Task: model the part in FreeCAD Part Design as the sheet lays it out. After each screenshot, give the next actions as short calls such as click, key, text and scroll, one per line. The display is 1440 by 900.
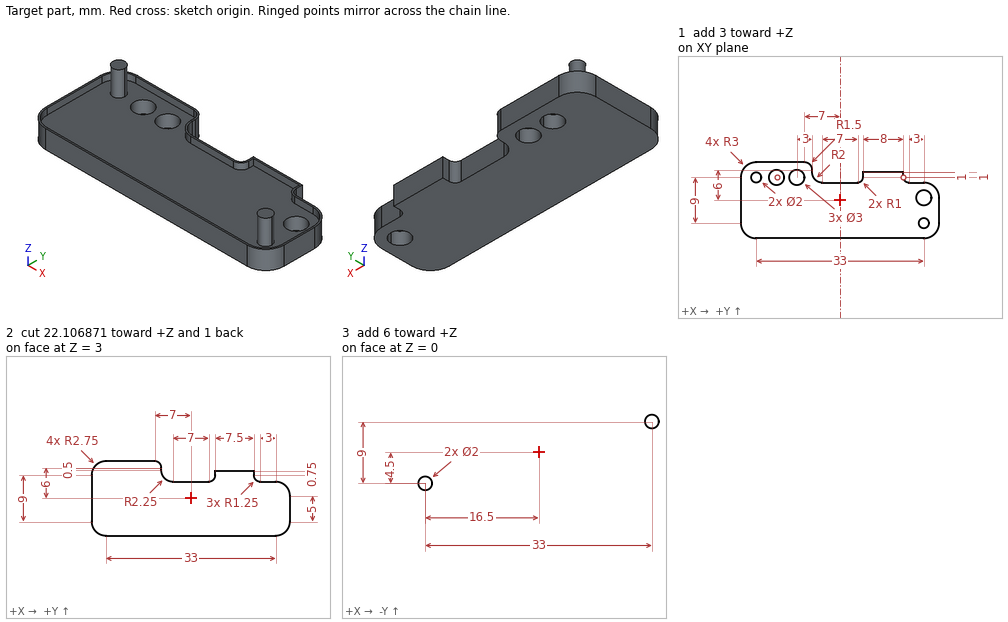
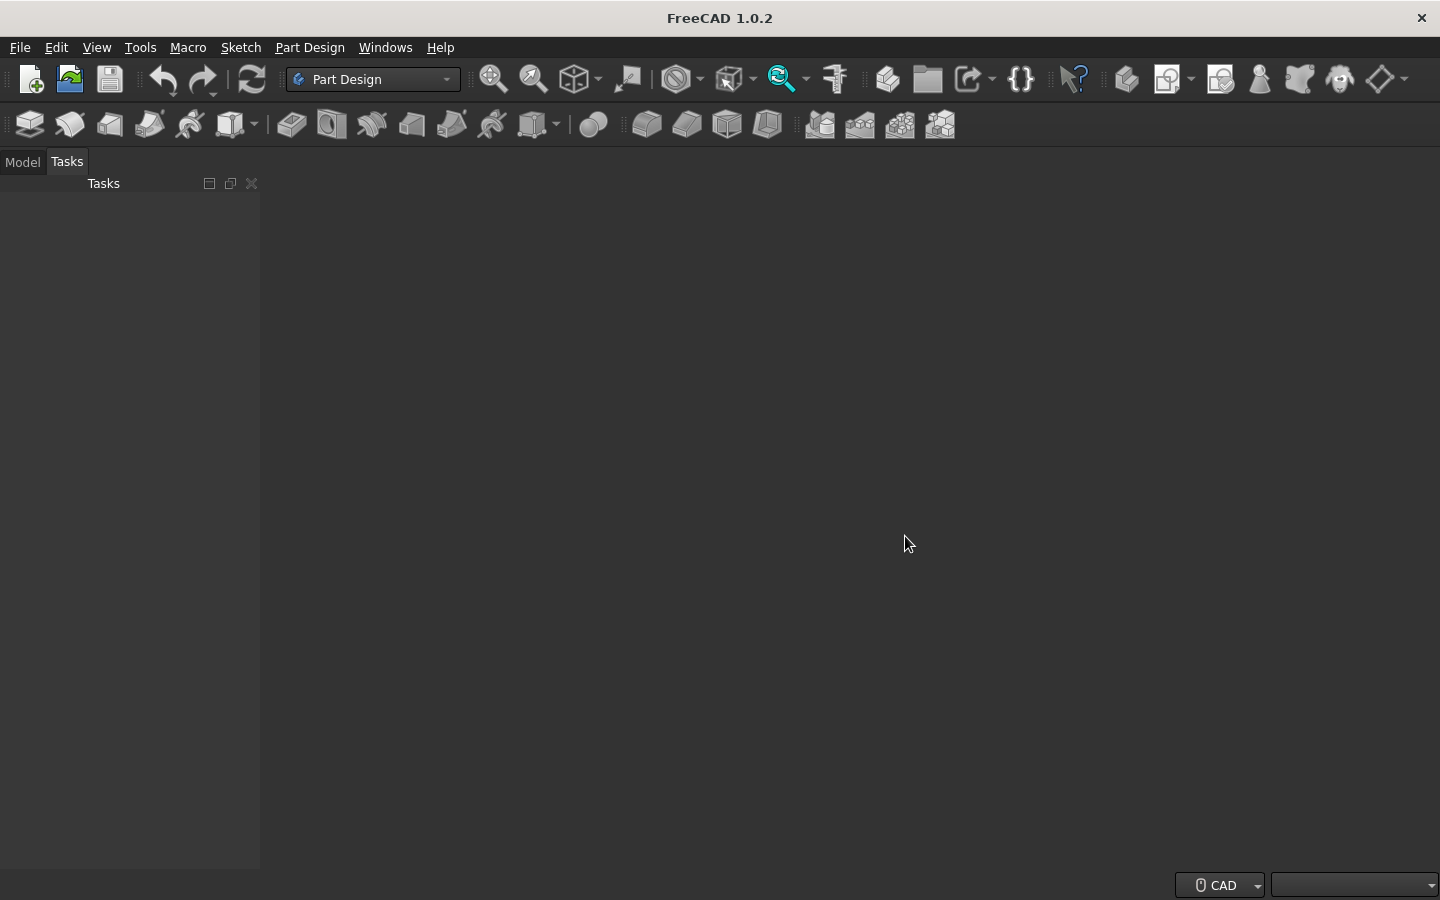
click(30, 80)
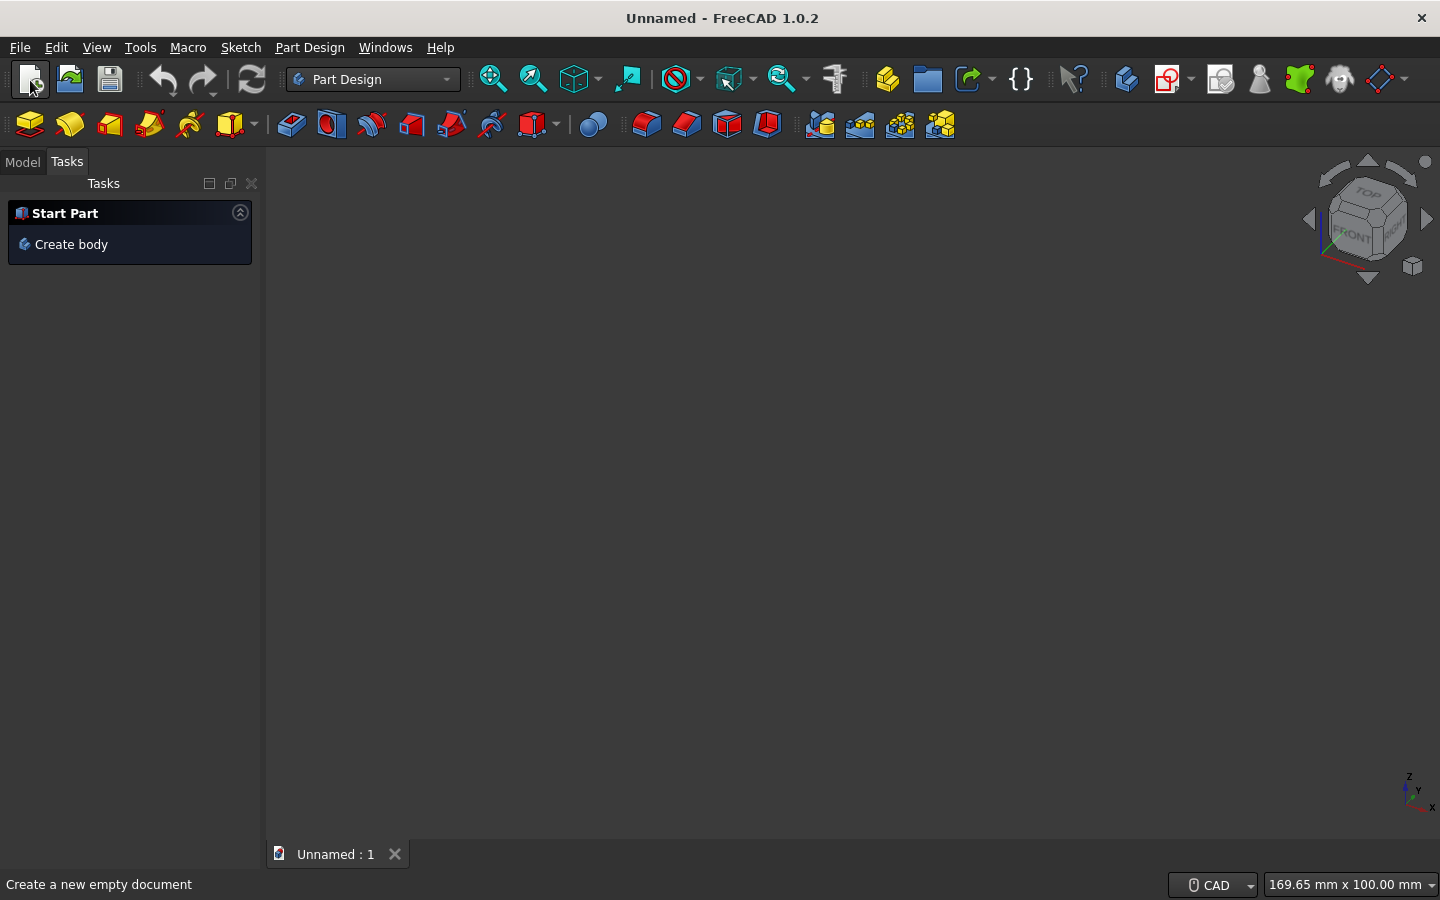
click(1168, 80)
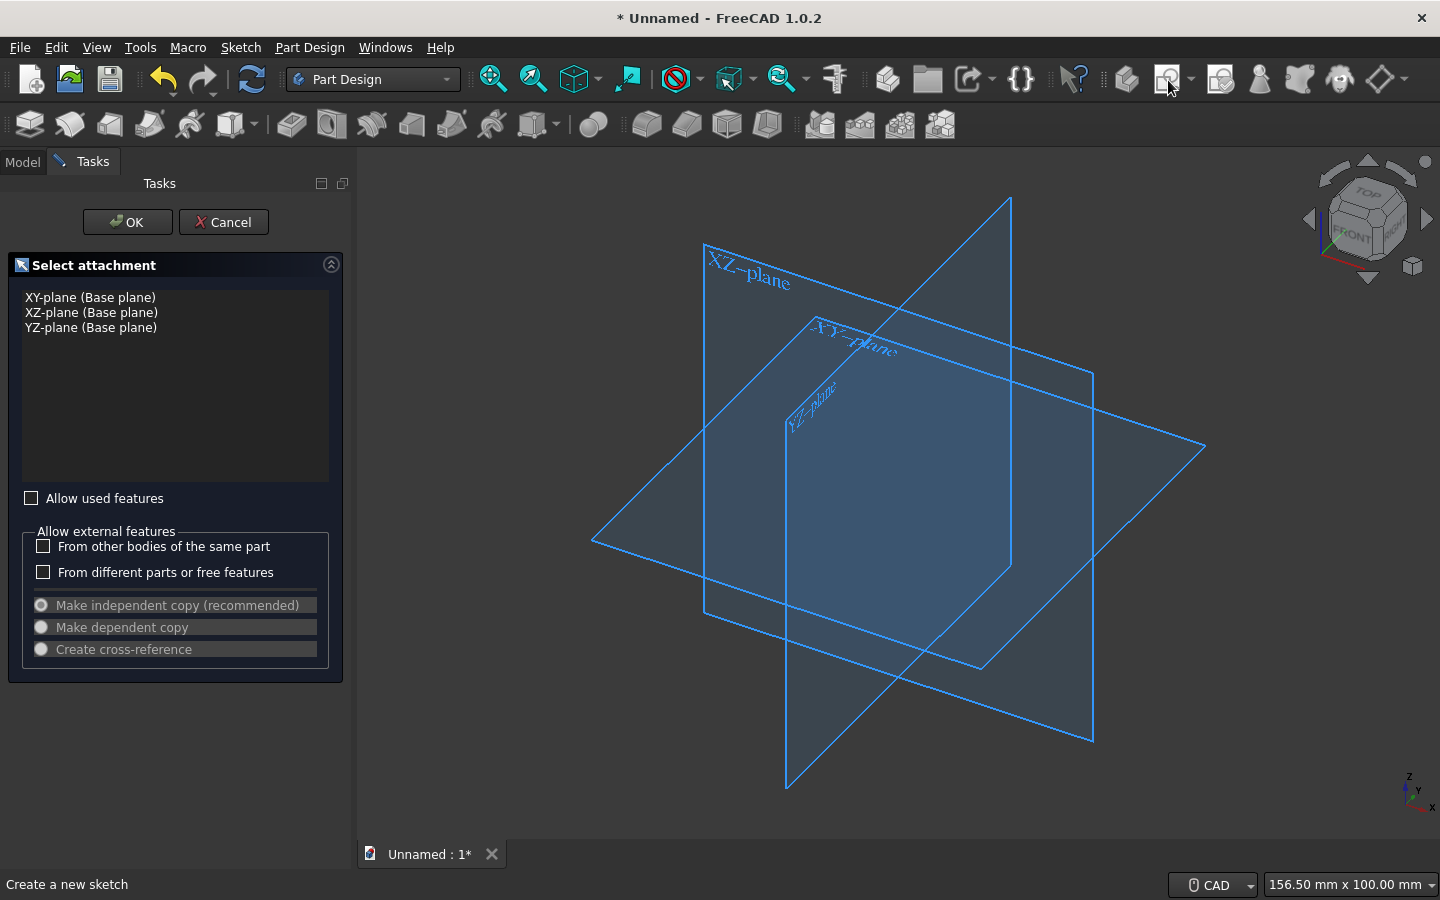
click(82, 298)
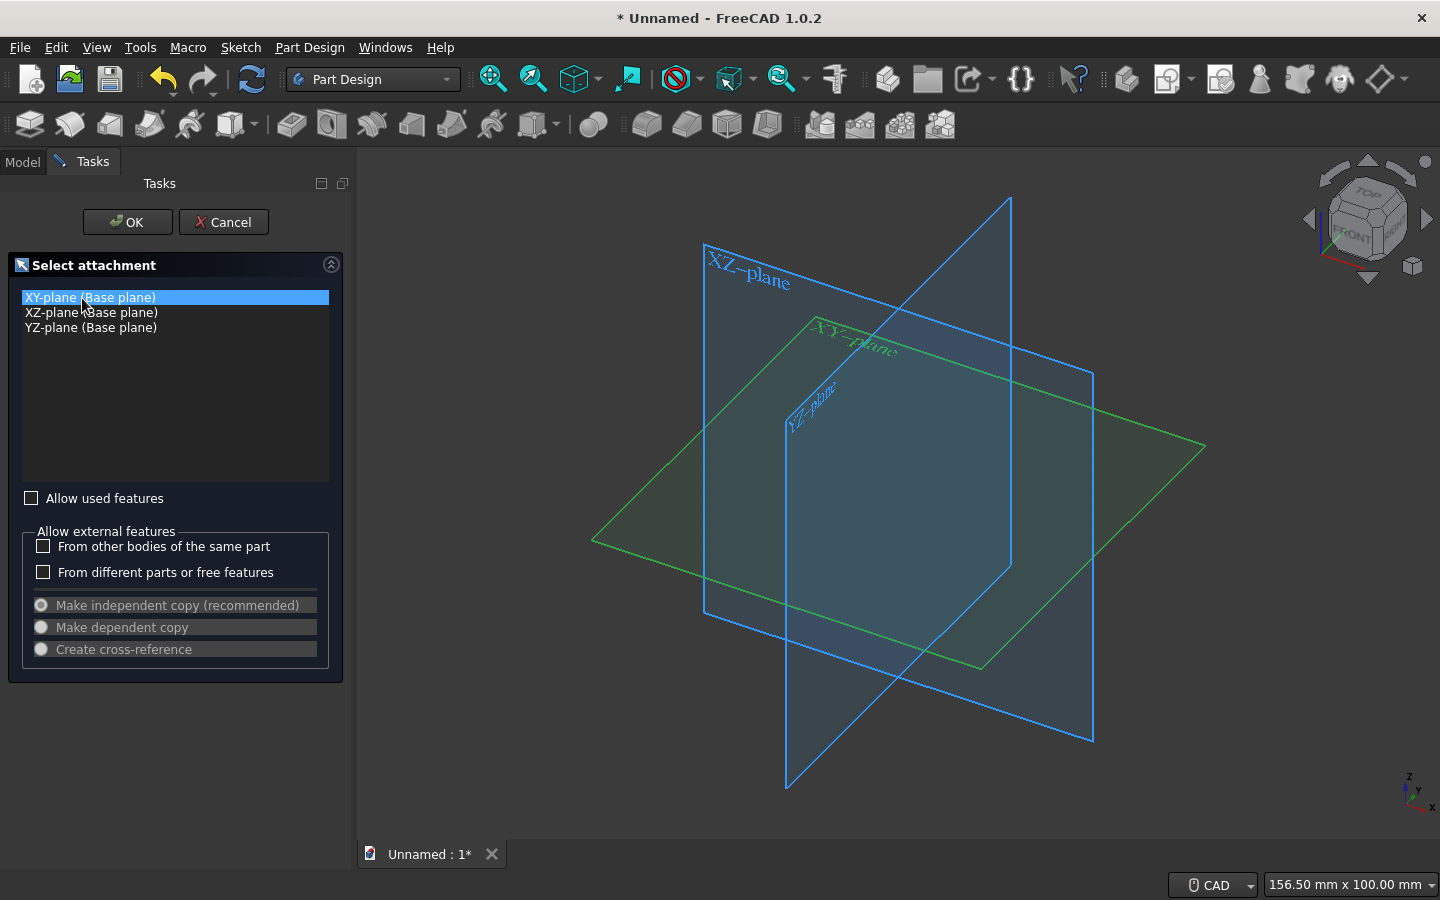
click(128, 222)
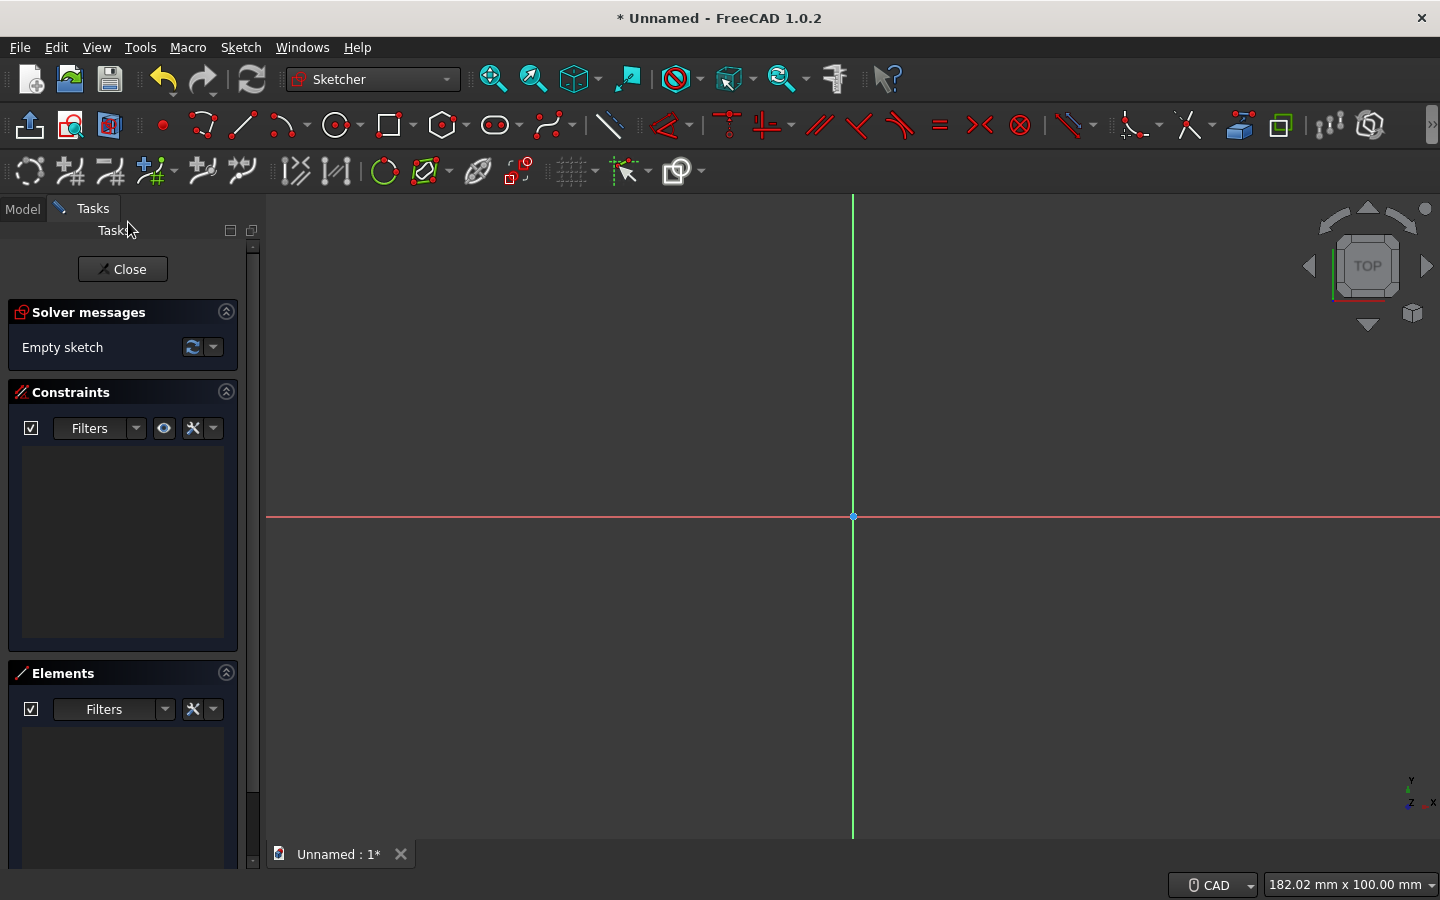
scroll(893, 516, up, 5)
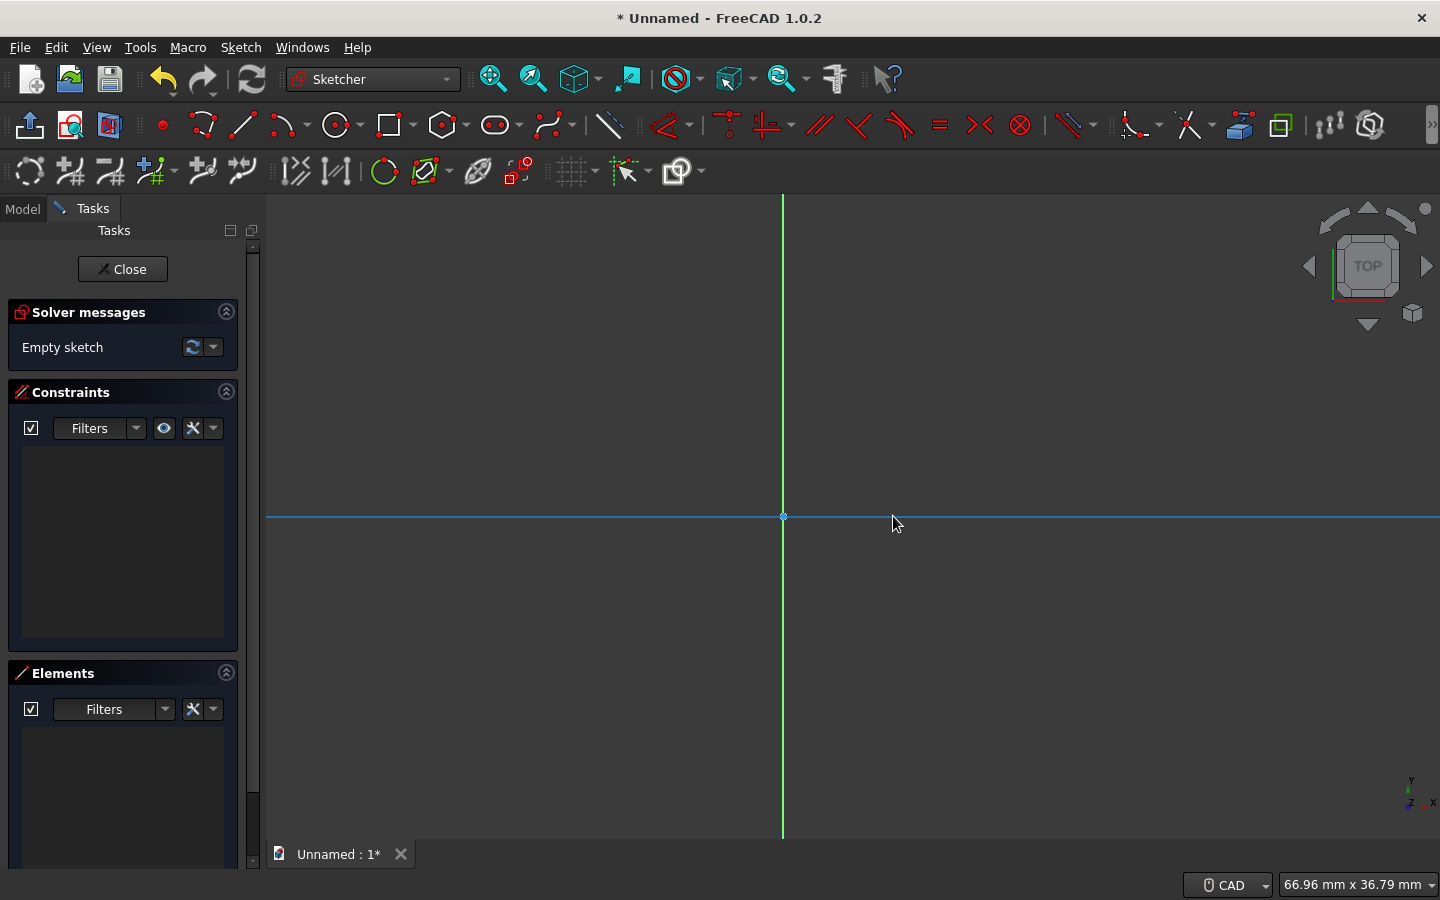
key(g)
key(l)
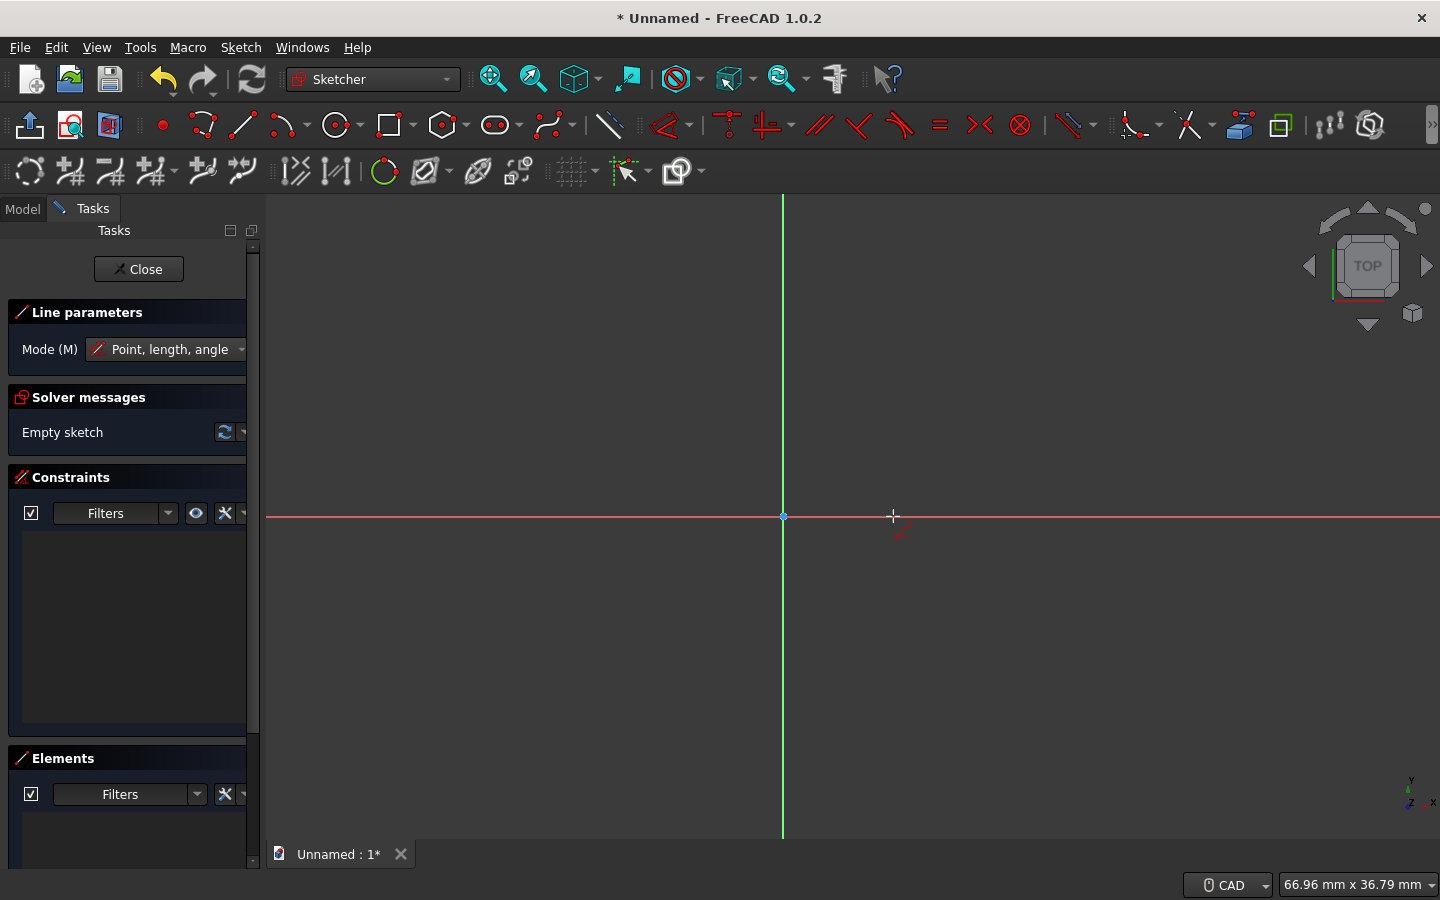
click(845, 455)
click(722, 455)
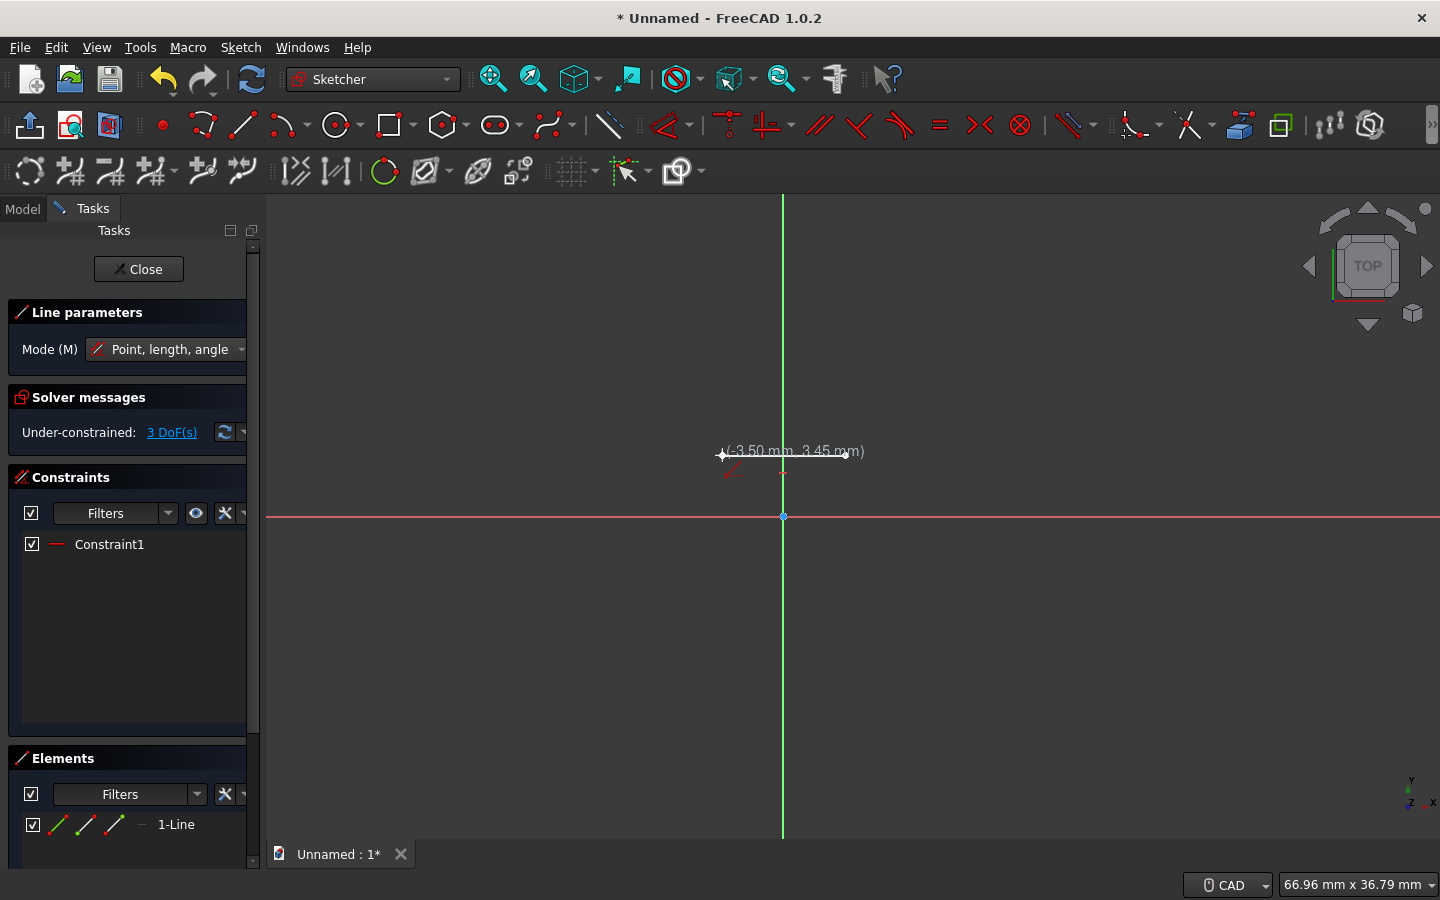
click(687, 420)